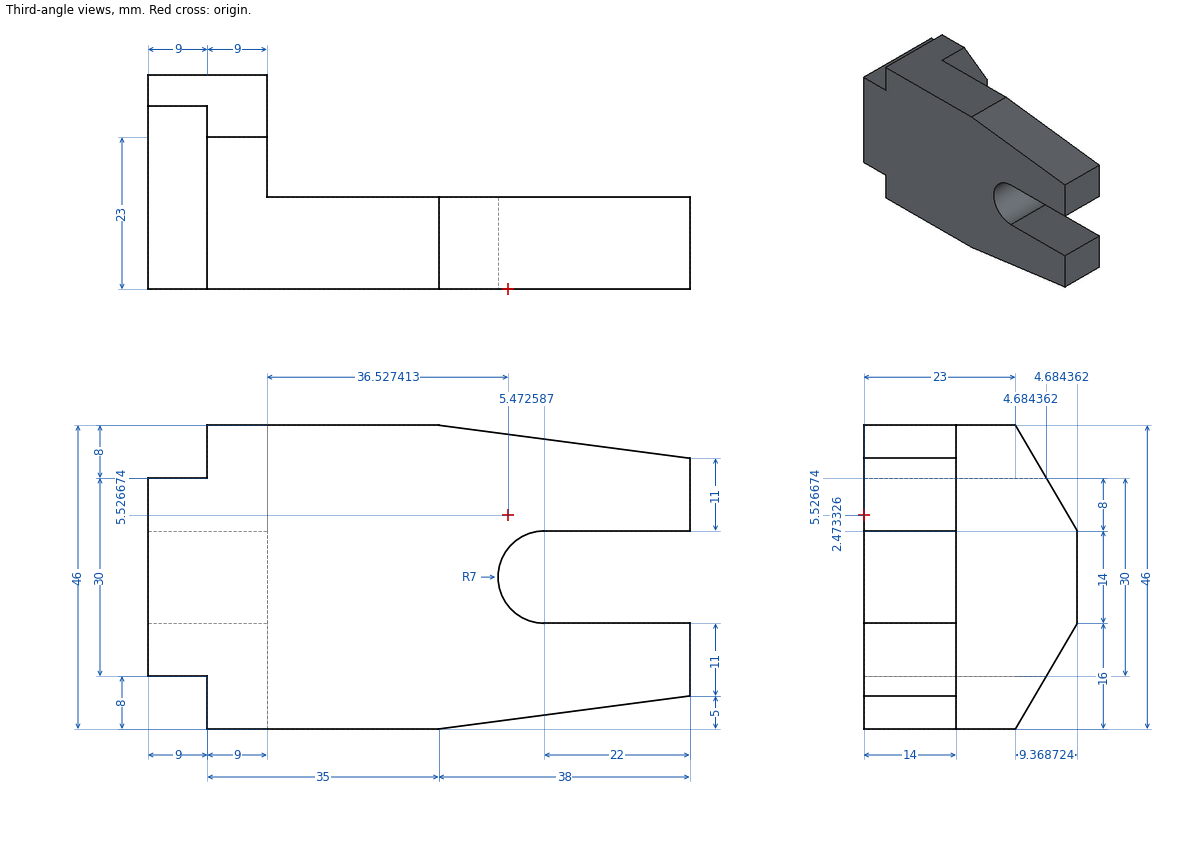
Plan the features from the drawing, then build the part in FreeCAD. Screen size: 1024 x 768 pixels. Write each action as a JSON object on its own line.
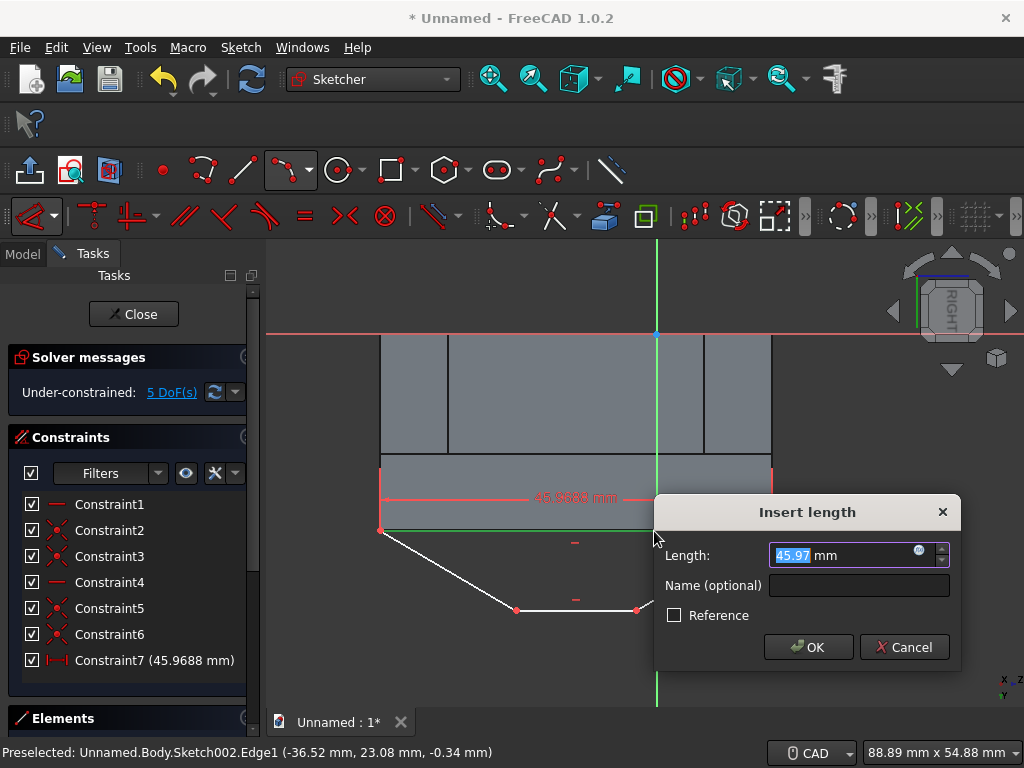
{"action": "type", "text": "46"}
{"action": "key", "text": "Return"}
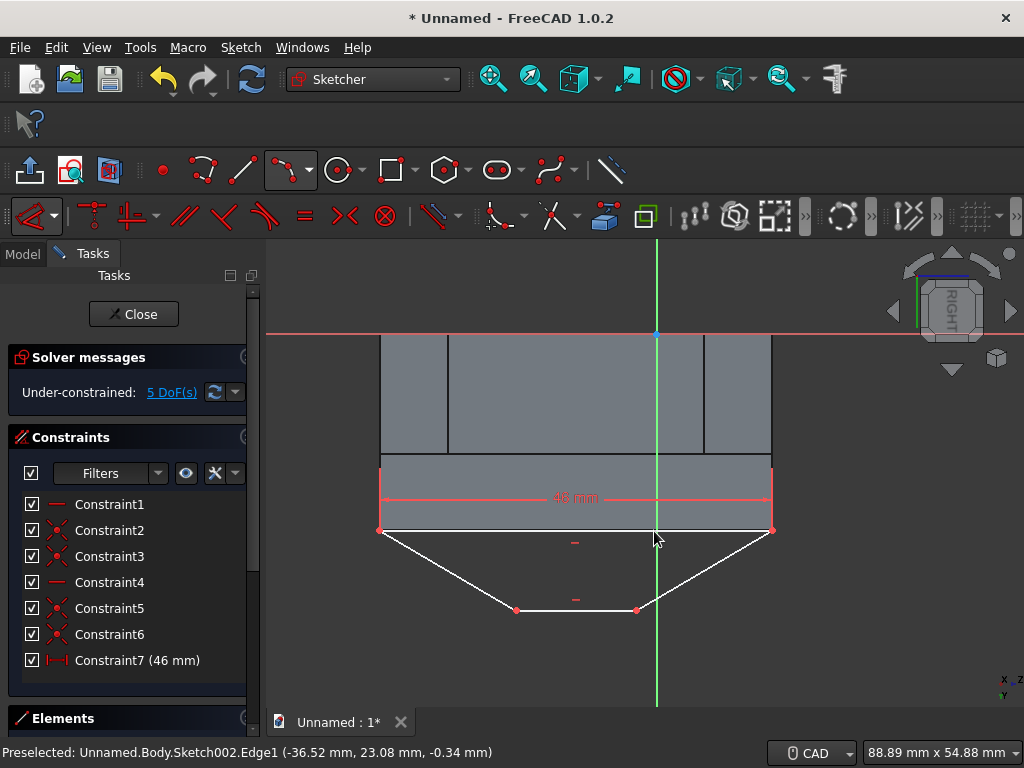
{"action": "left_click", "coordinate": [552, 611]}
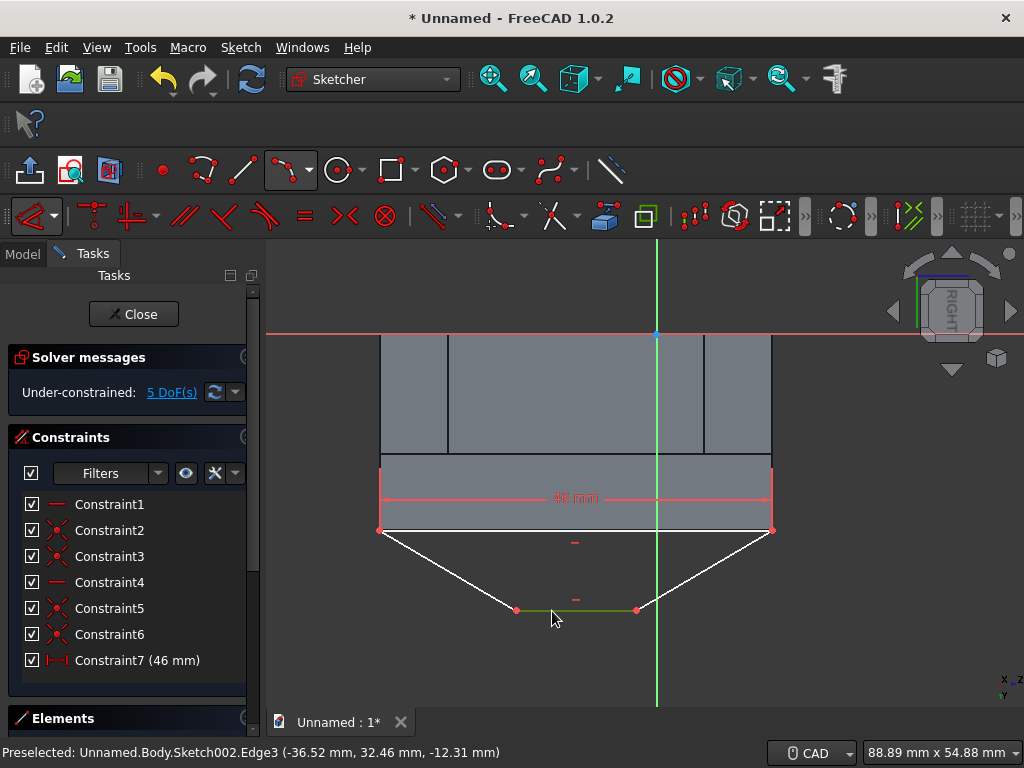
{"action": "key", "text": "l"}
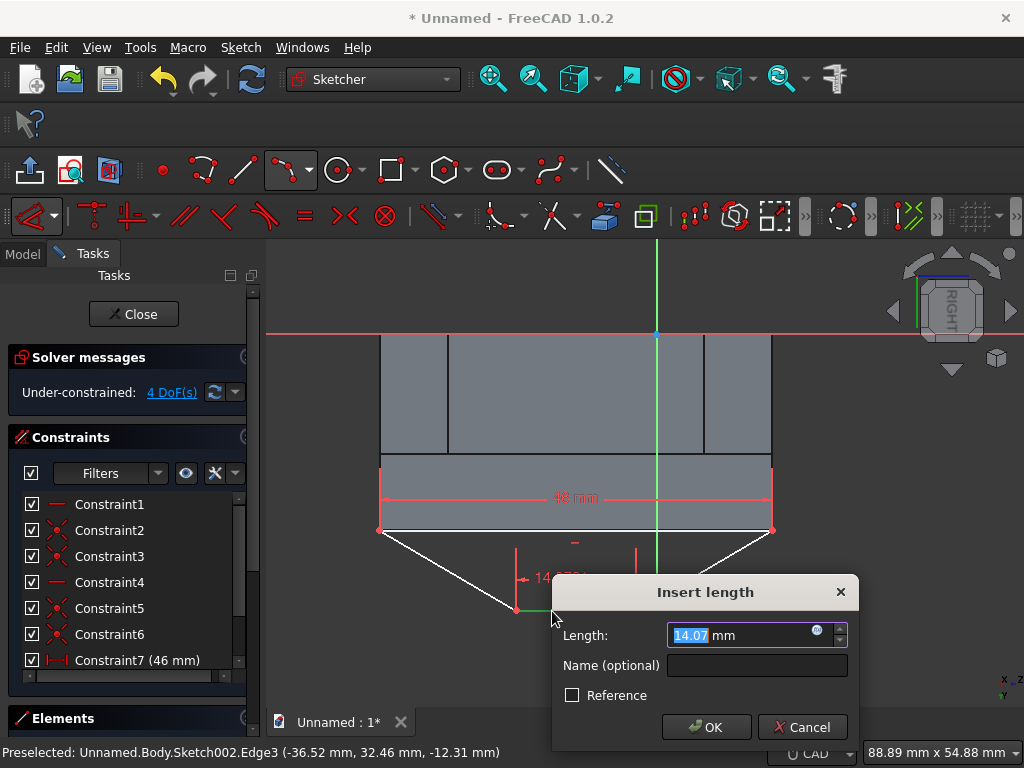
{"action": "type", "text": "14"}
{"action": "key", "text": "Return"}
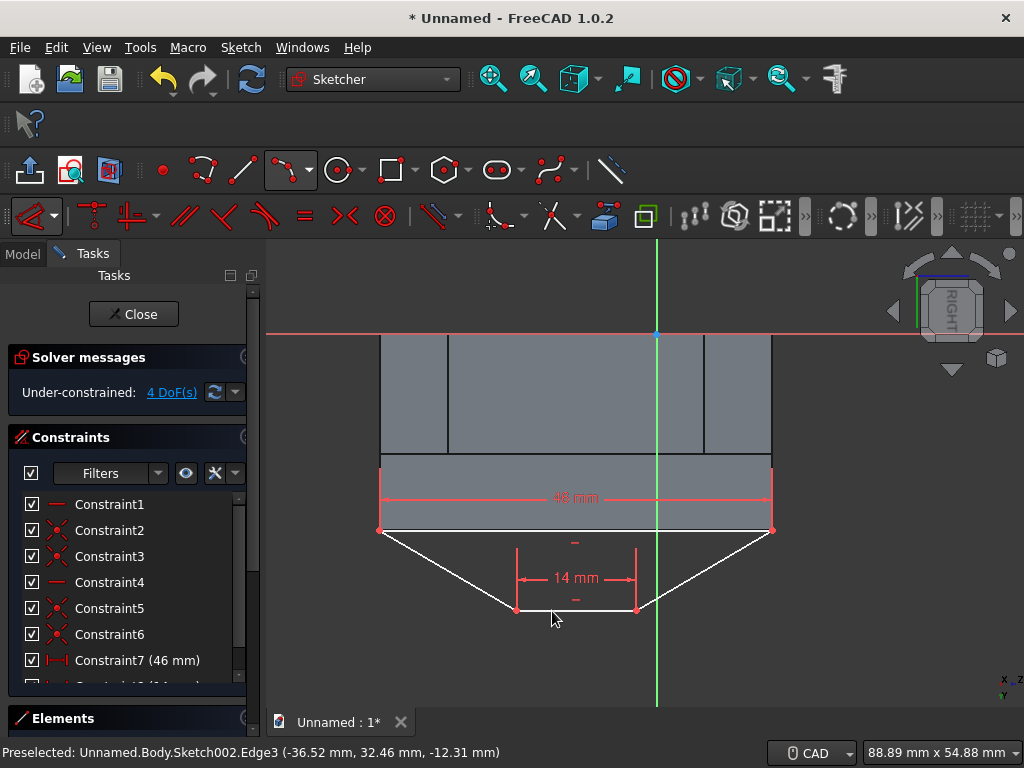
{"action": "left_click", "coordinate": [772, 531]}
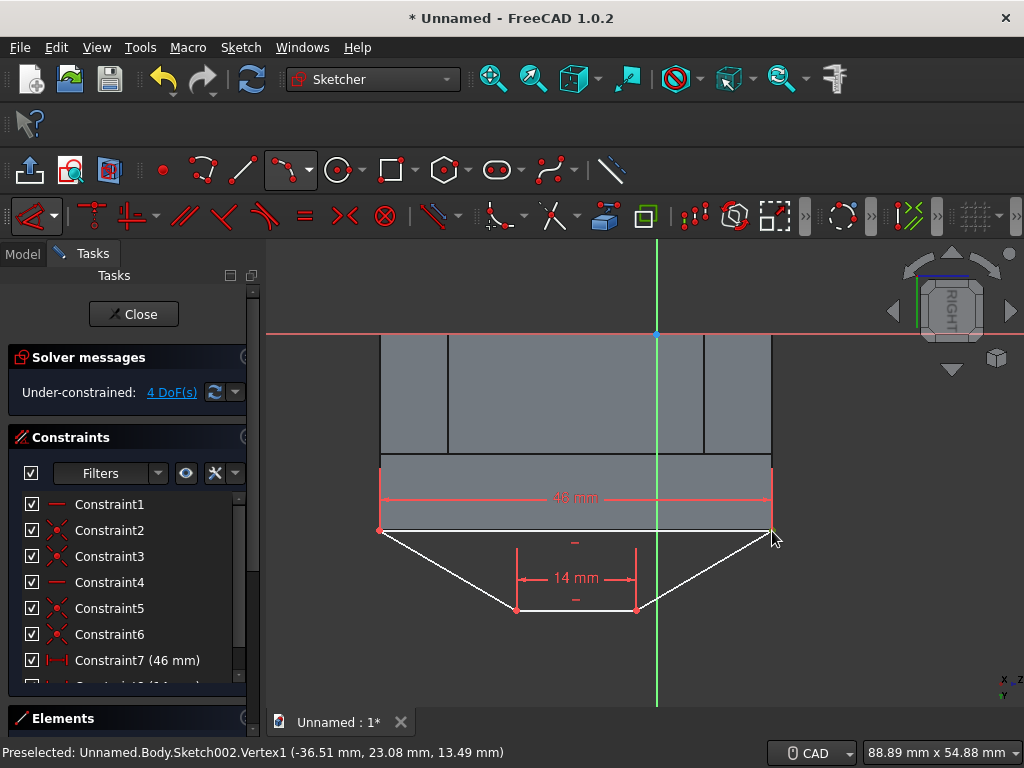
{"action": "left_click", "coordinate": [56, 216]}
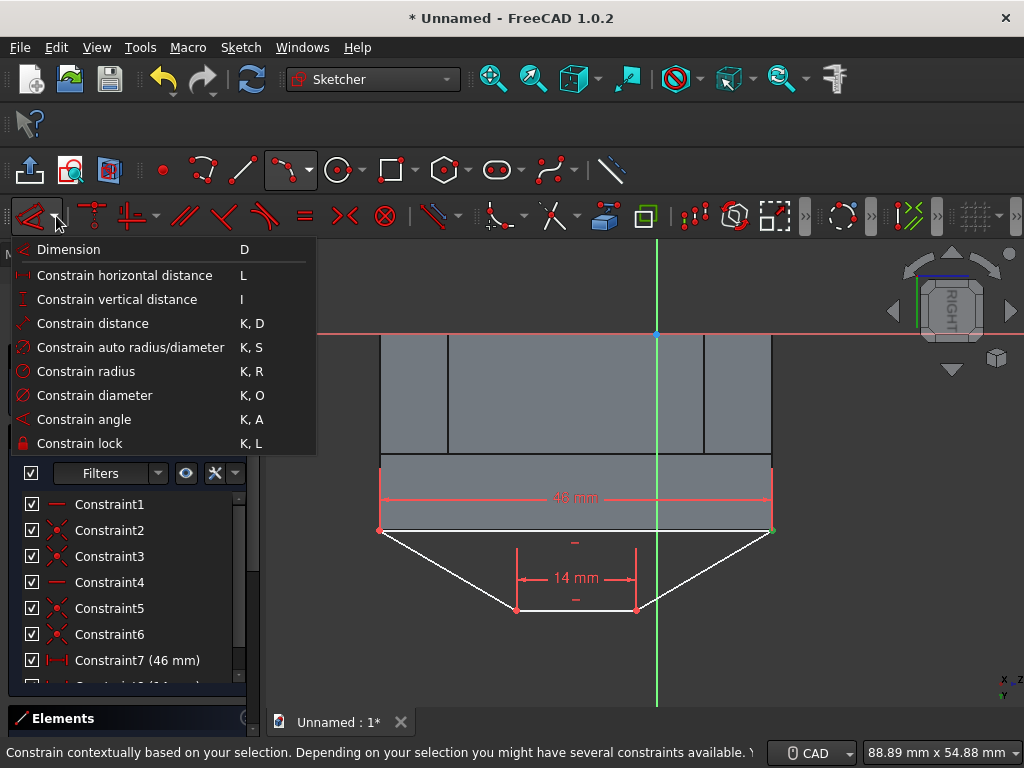
{"action": "left_click", "coordinate": [164, 299]}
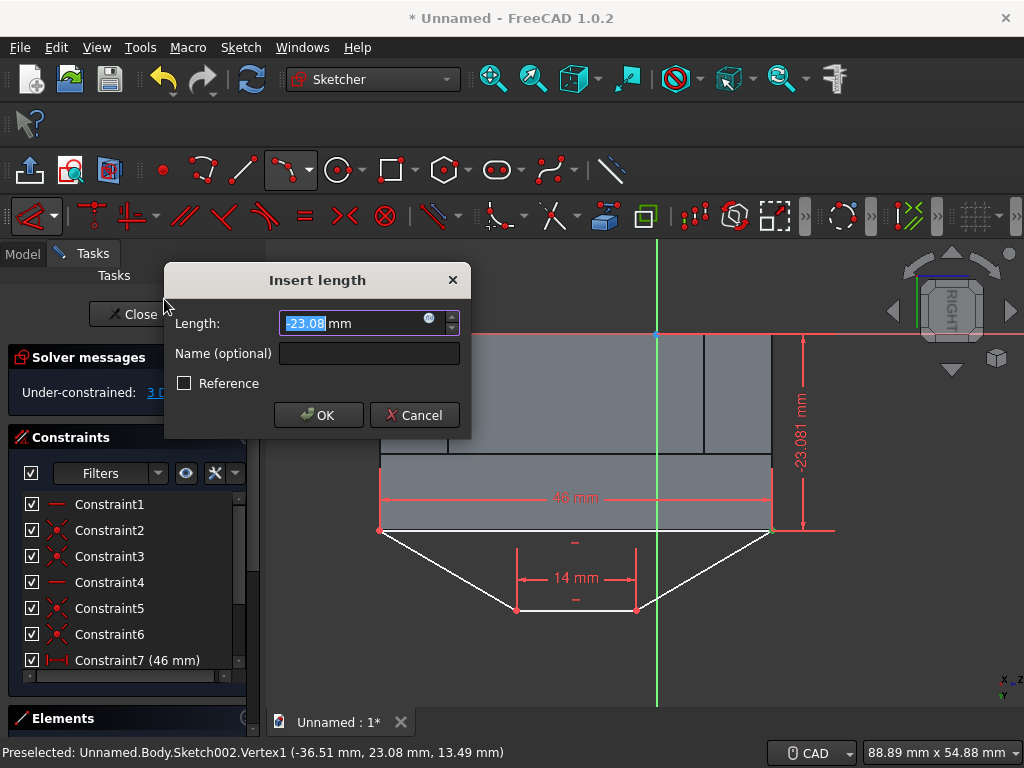
{"action": "type", "text": "-23"}
{"action": "key", "text": "Return"}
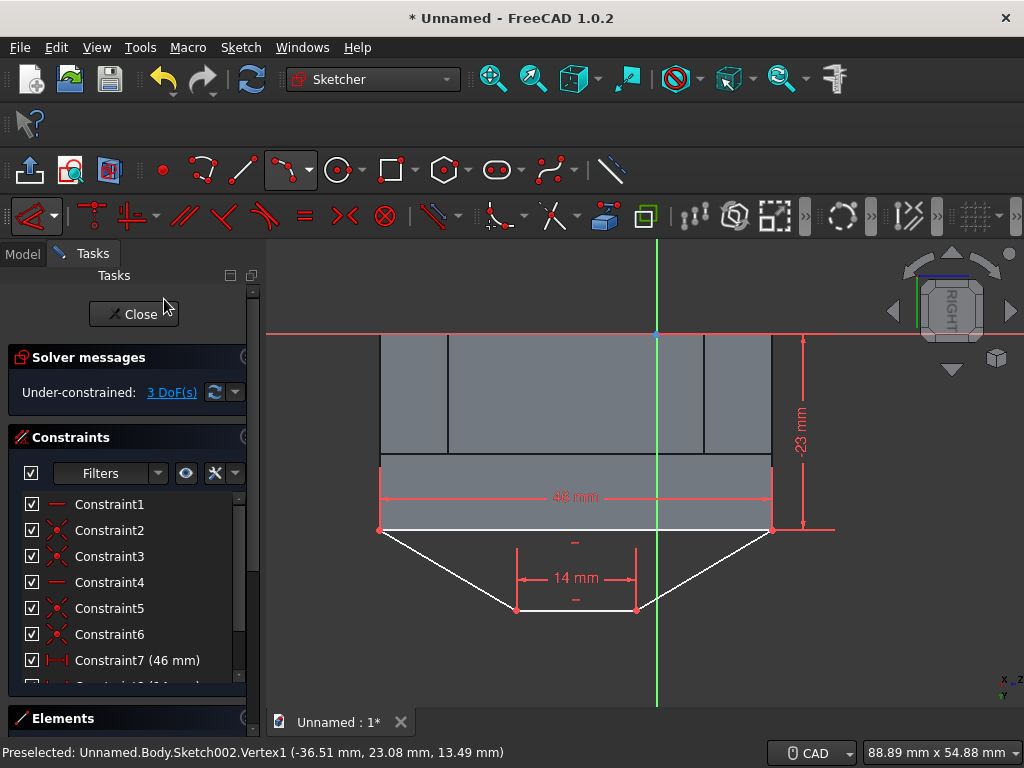
{"action": "left_click", "coordinate": [421, 555]}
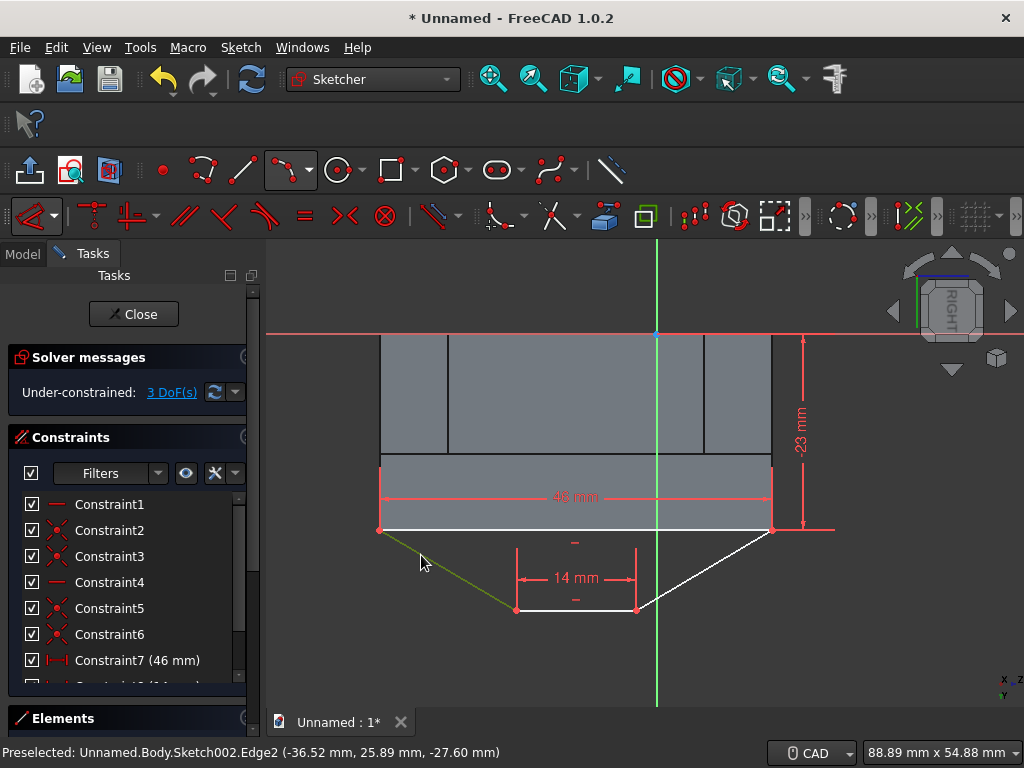
{"action": "left_click", "coordinate": [56, 216]}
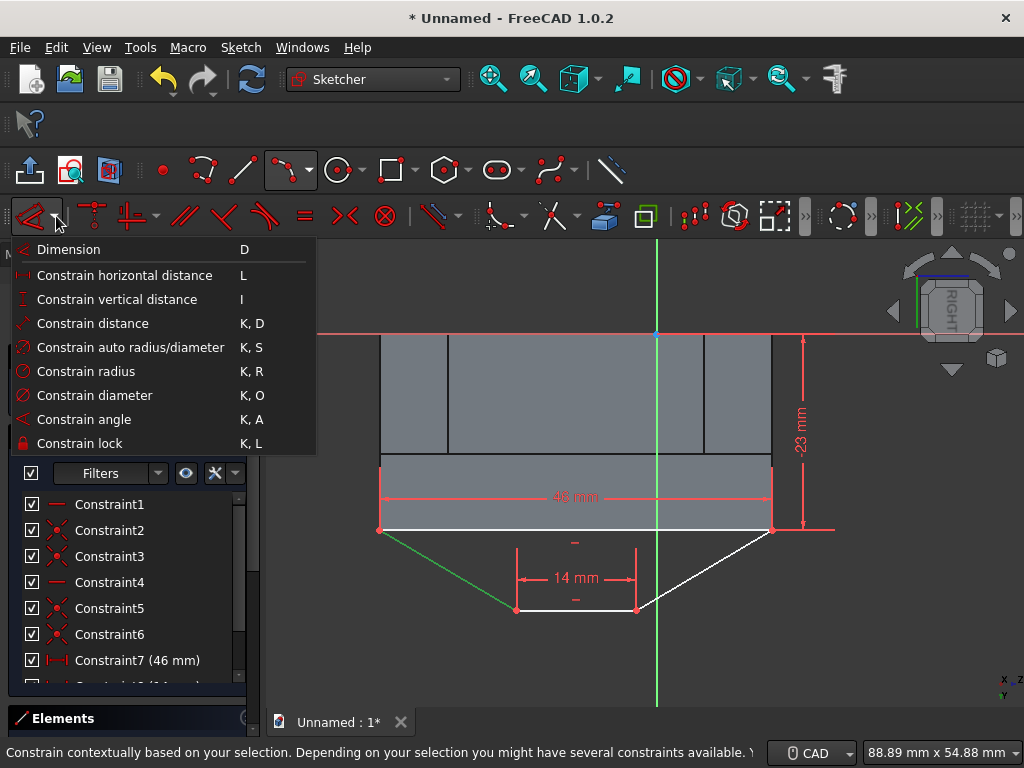
{"action": "left_click", "coordinate": [164, 275]}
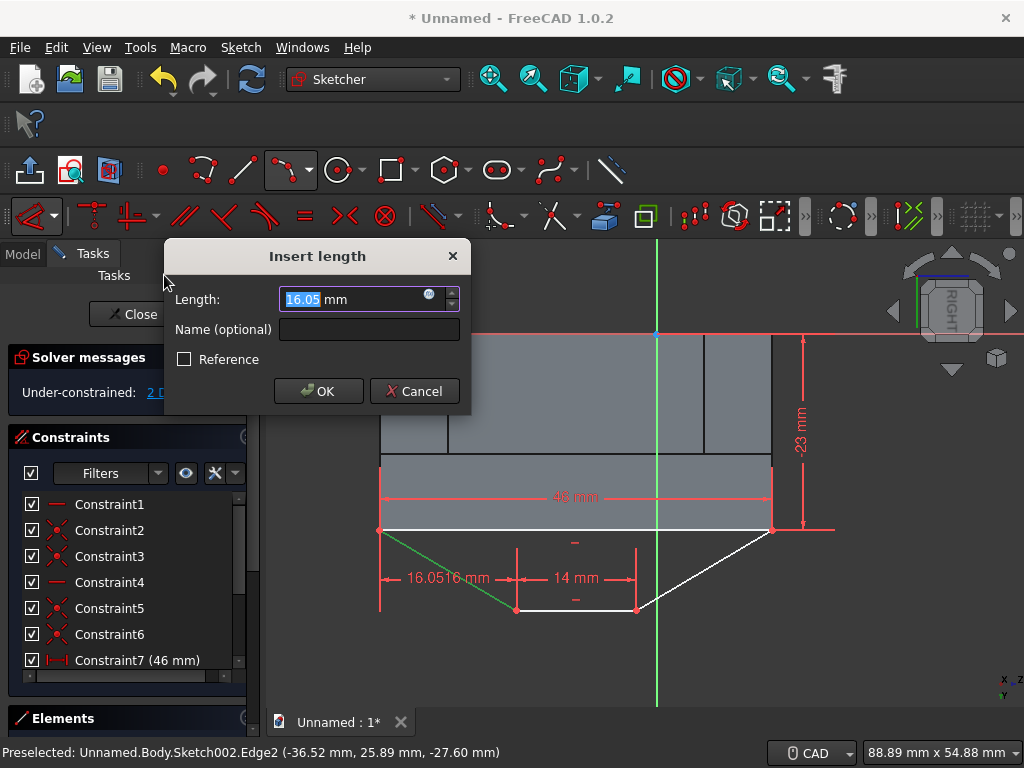
{"action": "type", "text": "16"}
{"action": "key", "text": "Return"}